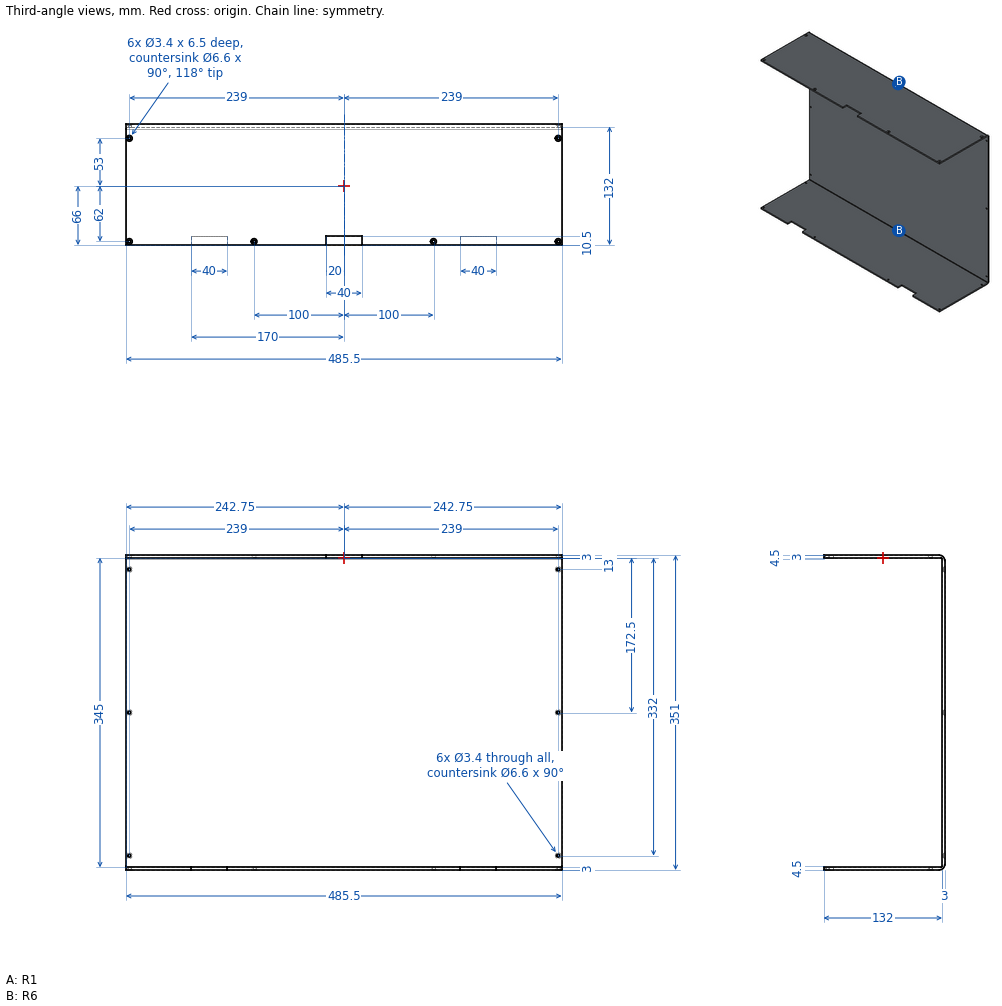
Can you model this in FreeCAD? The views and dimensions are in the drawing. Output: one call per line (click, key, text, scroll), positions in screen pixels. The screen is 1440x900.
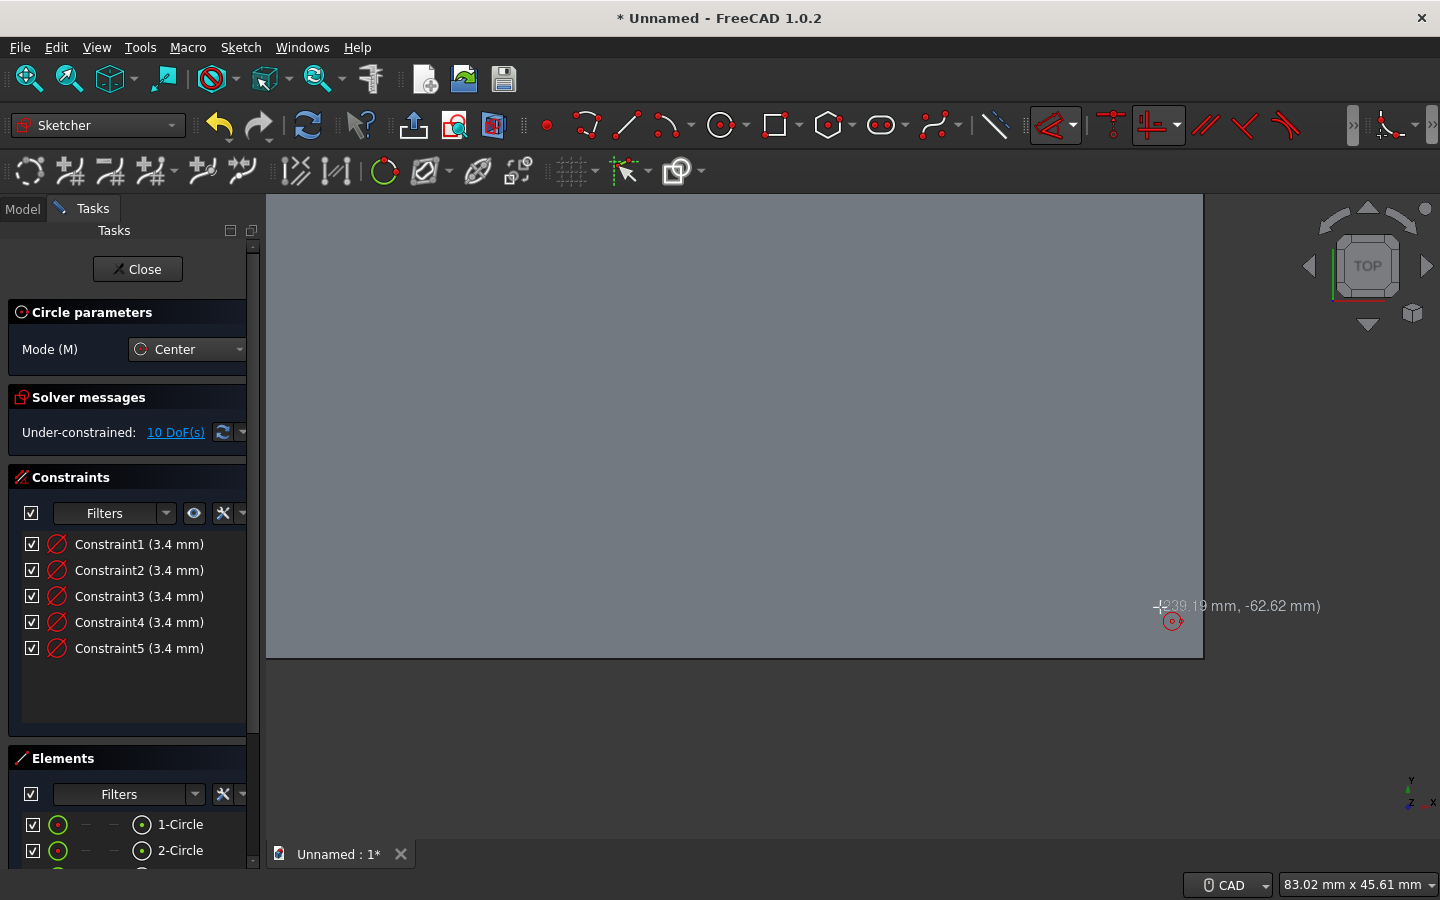
scroll(1160, 607, down, 11)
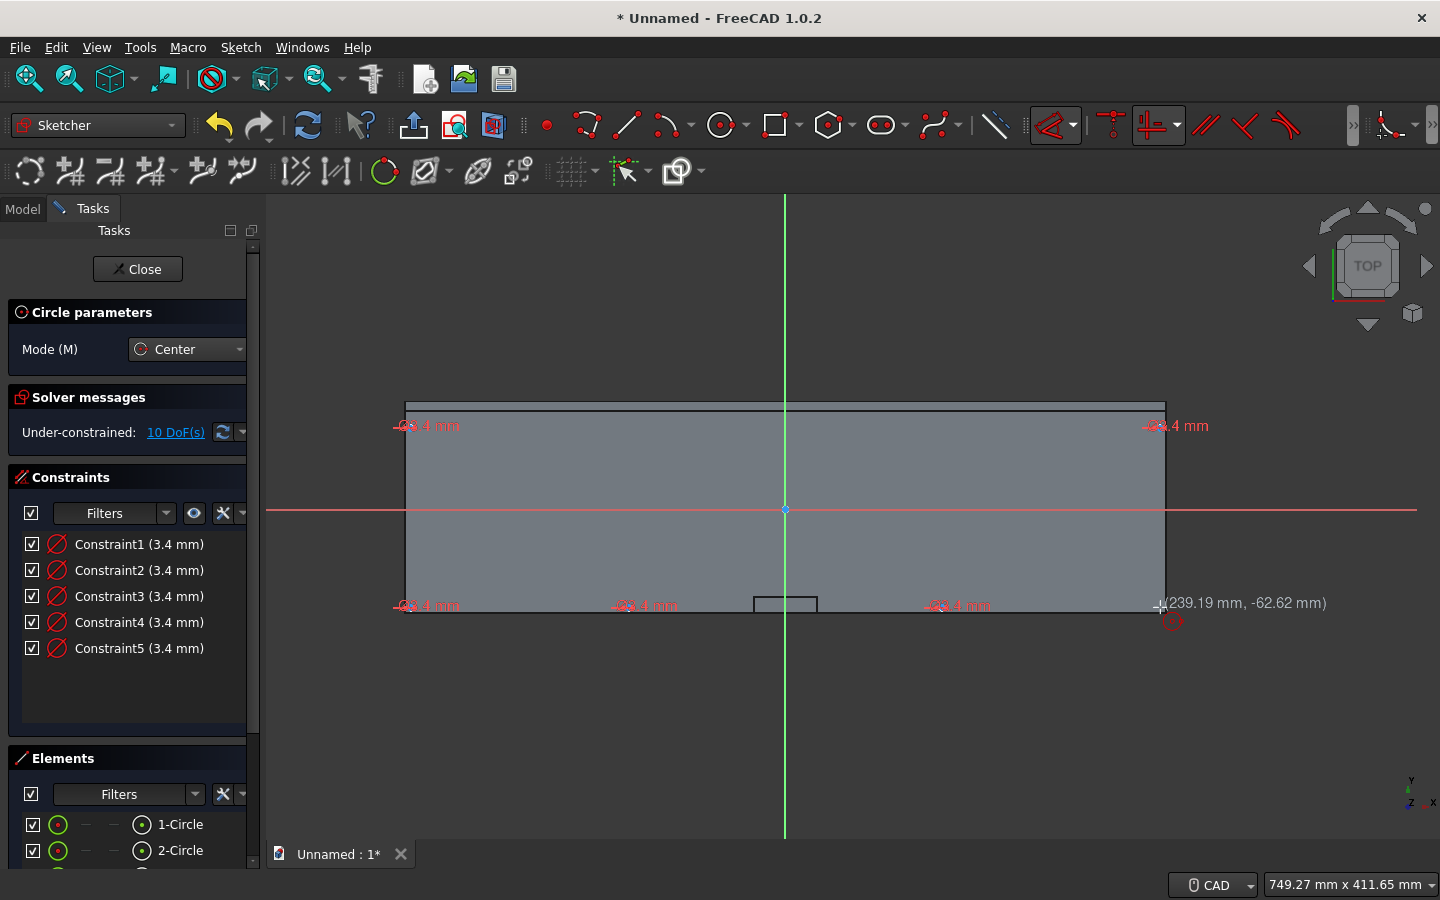
click(1160, 607)
move(1162, 605)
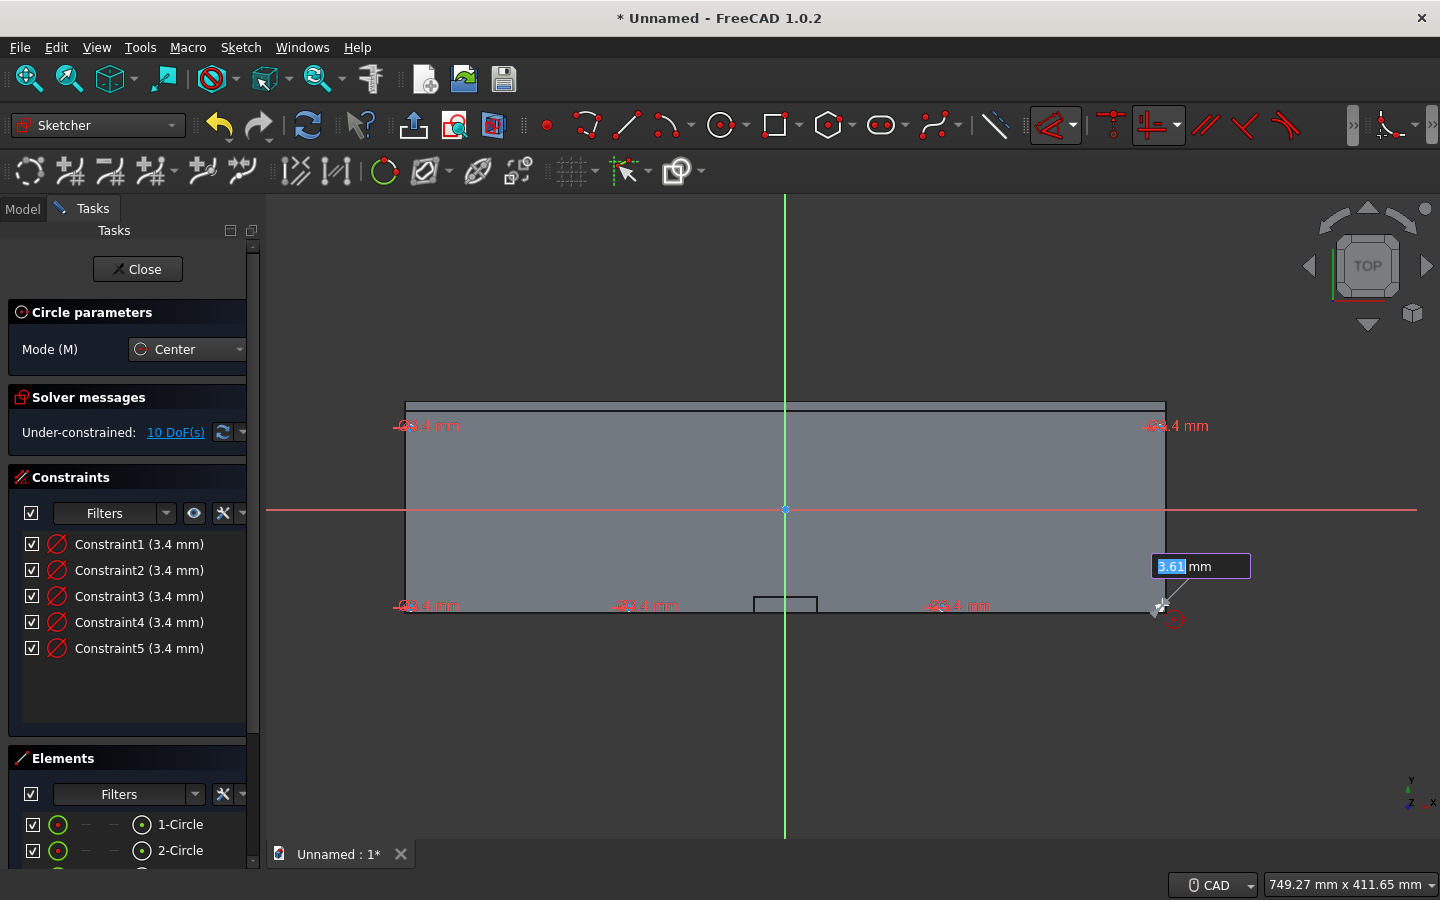
text(3.4)
key(Return)
key(Escape)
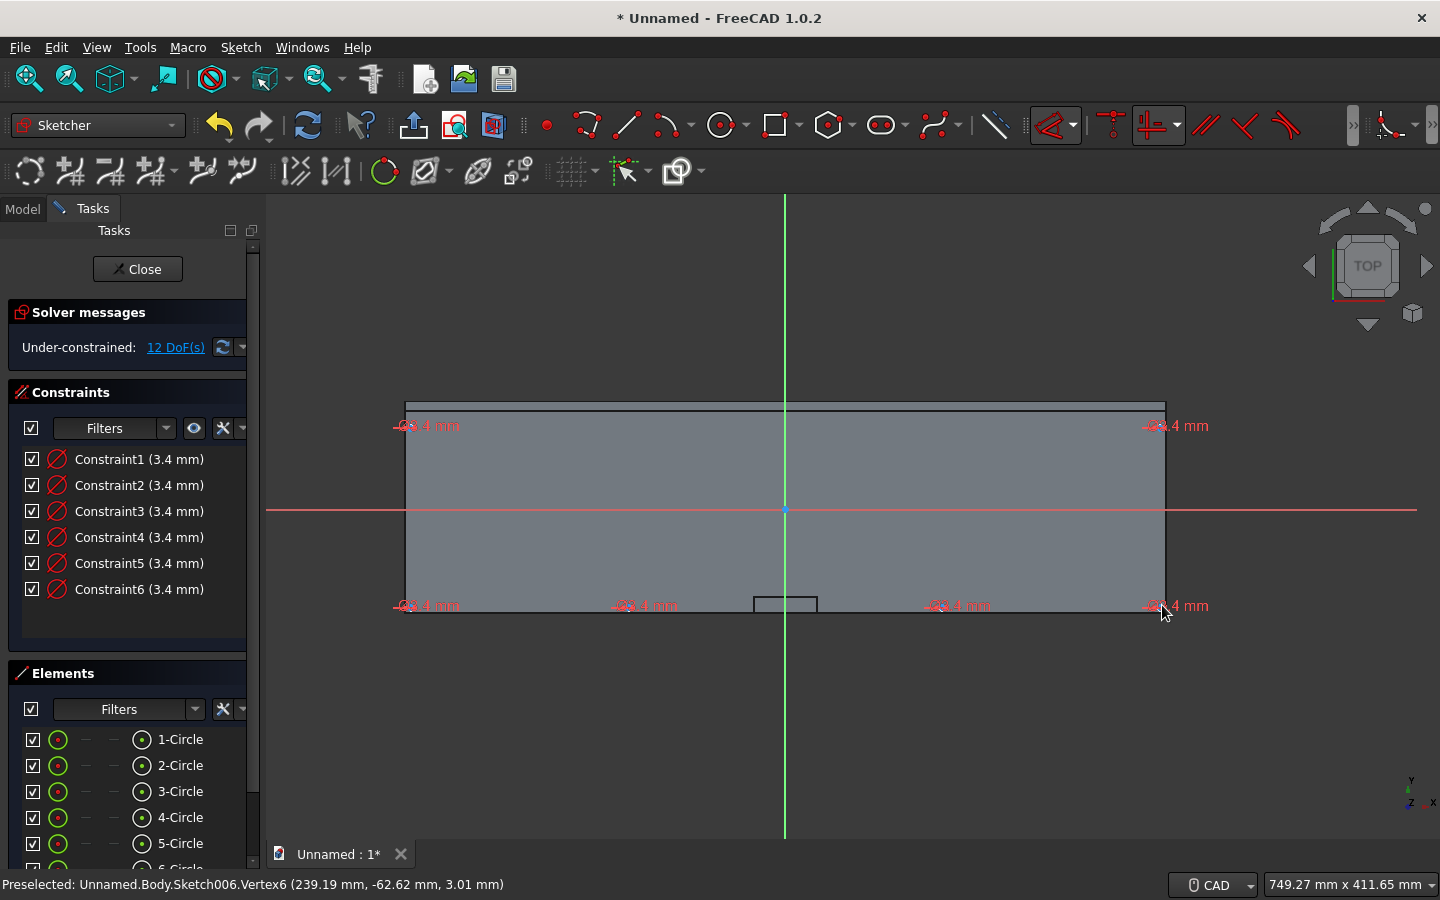
click(411, 428)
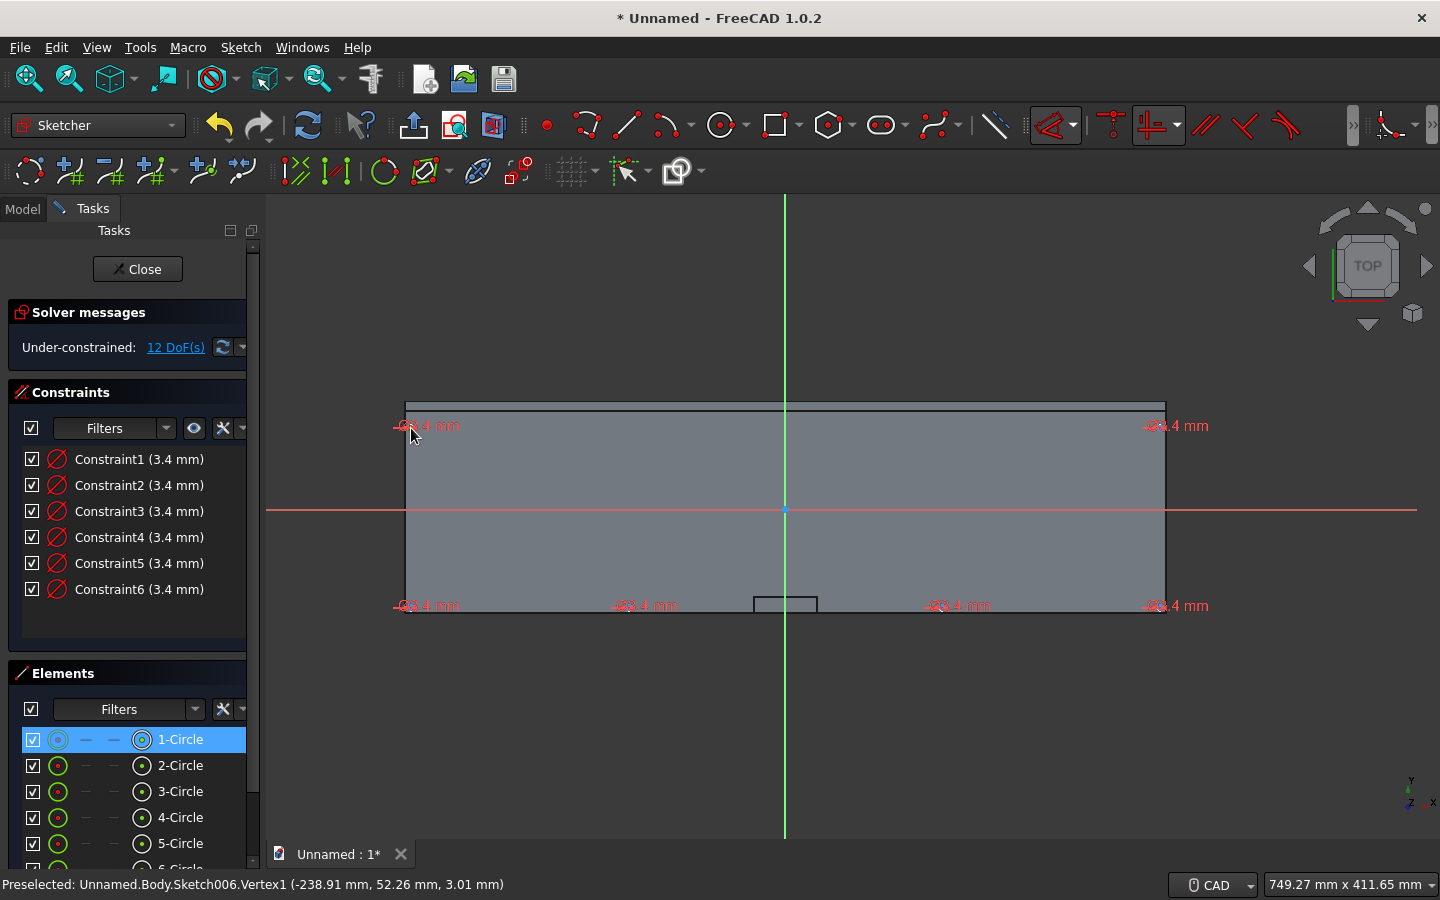
click(411, 608)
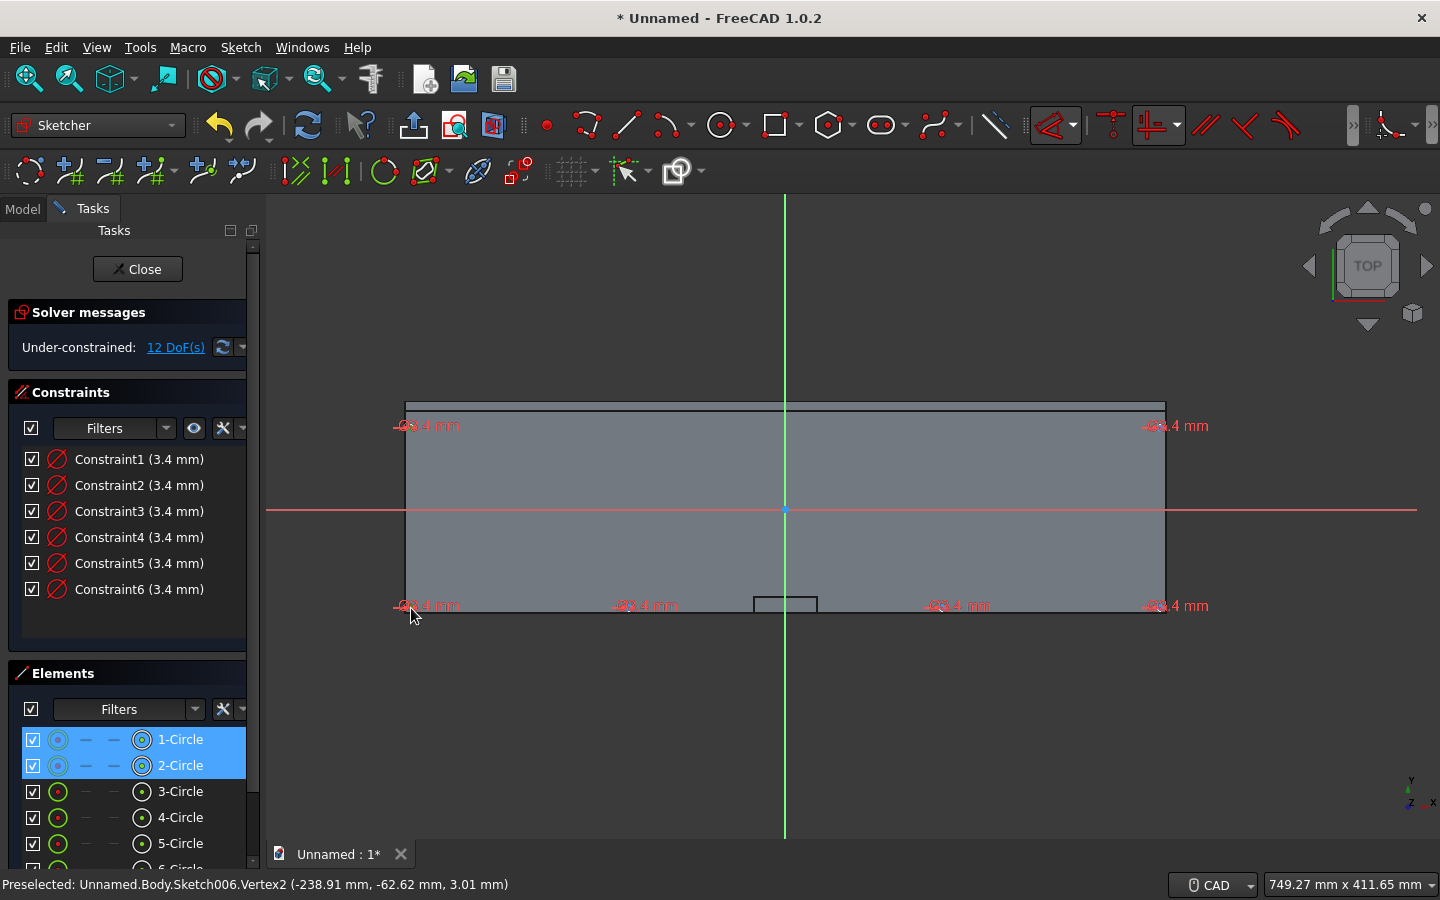
click(1180, 126)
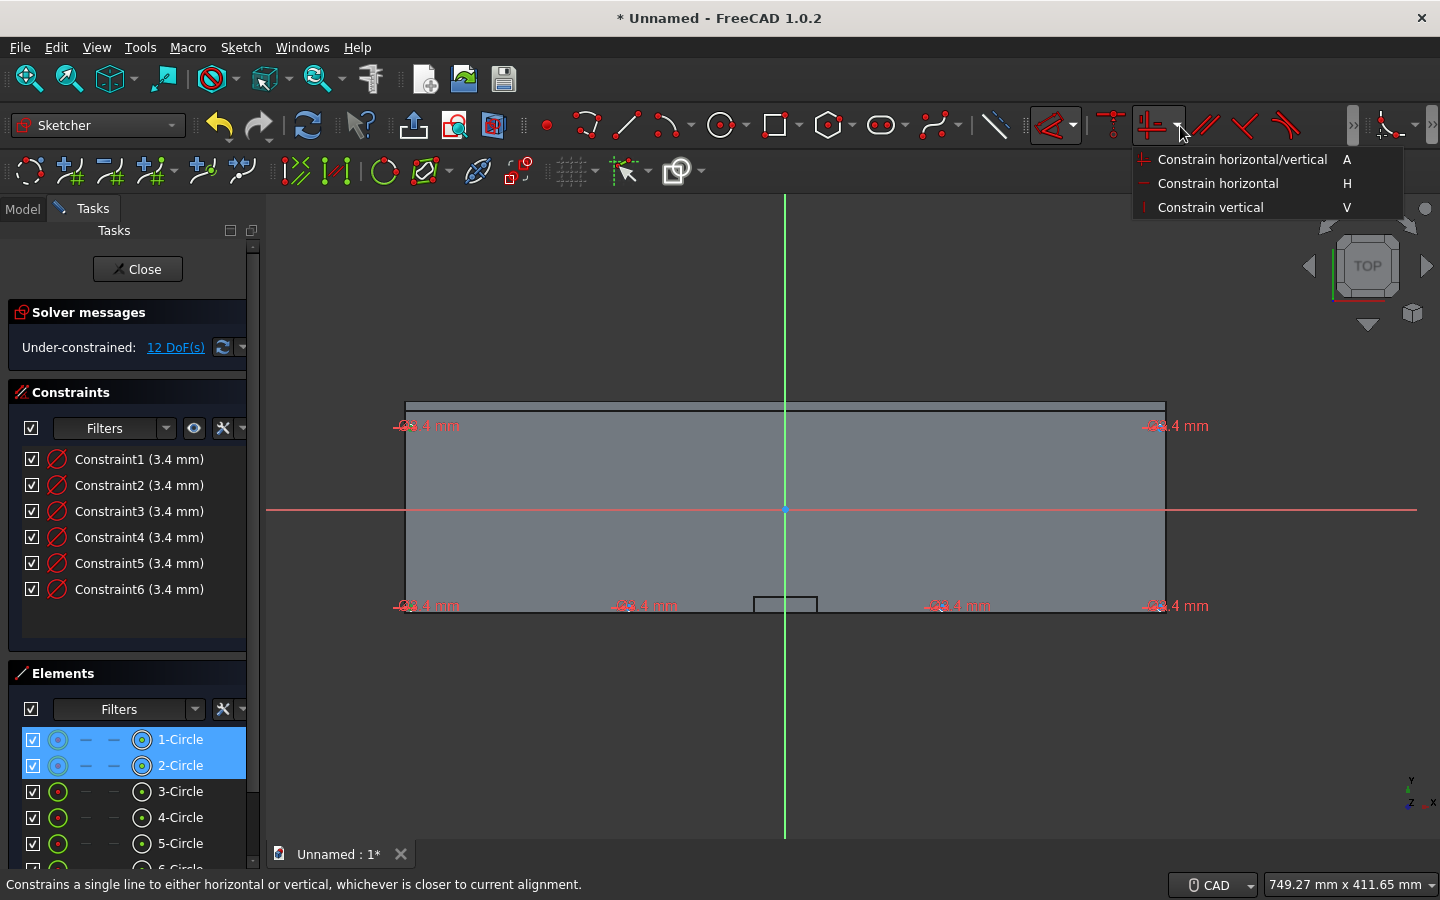
click(1268, 207)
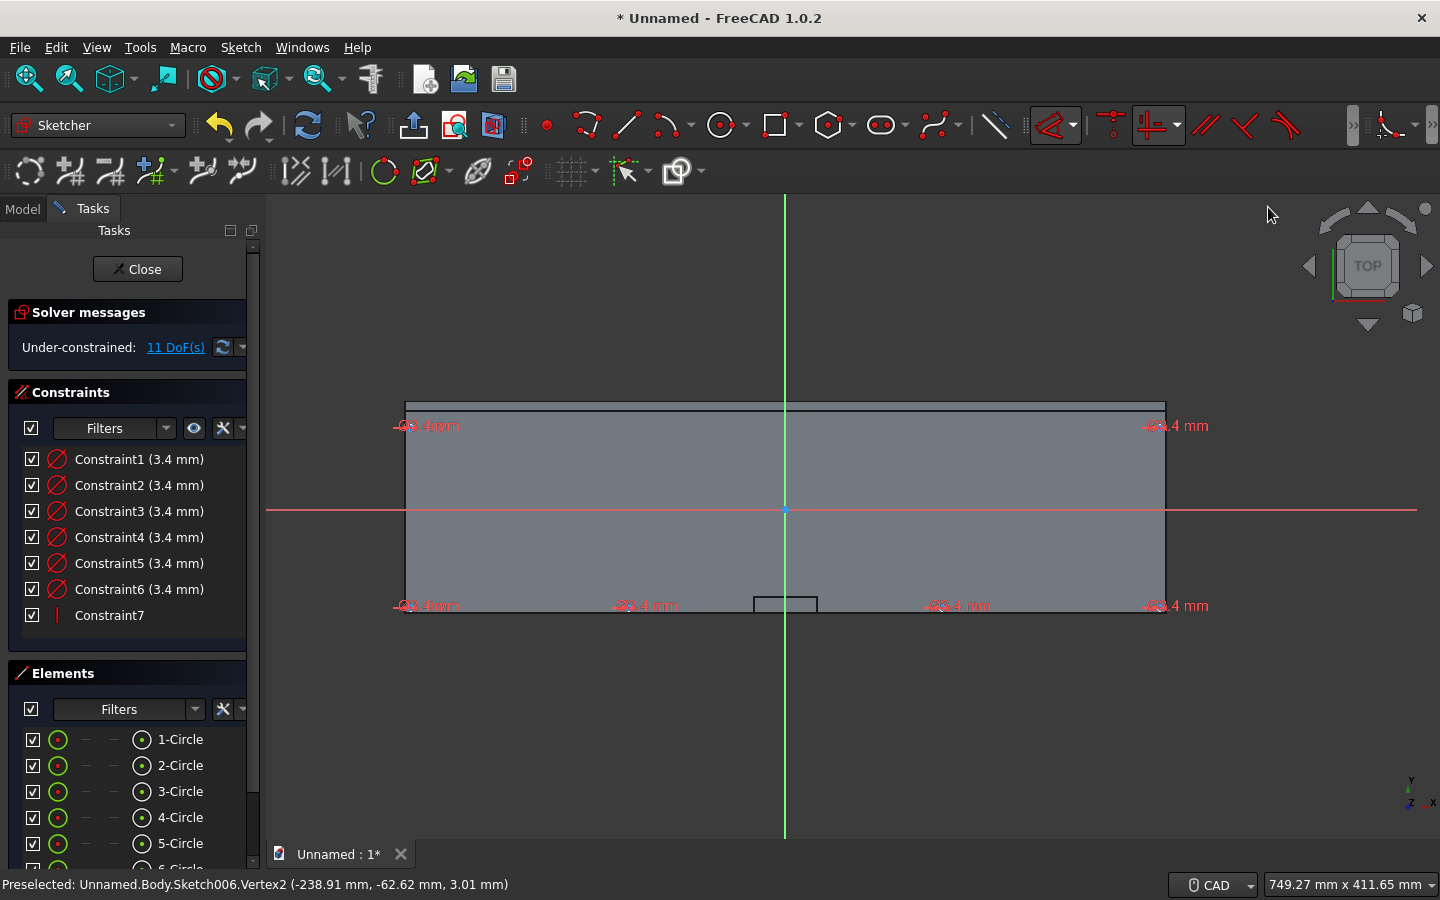
click(411, 608)